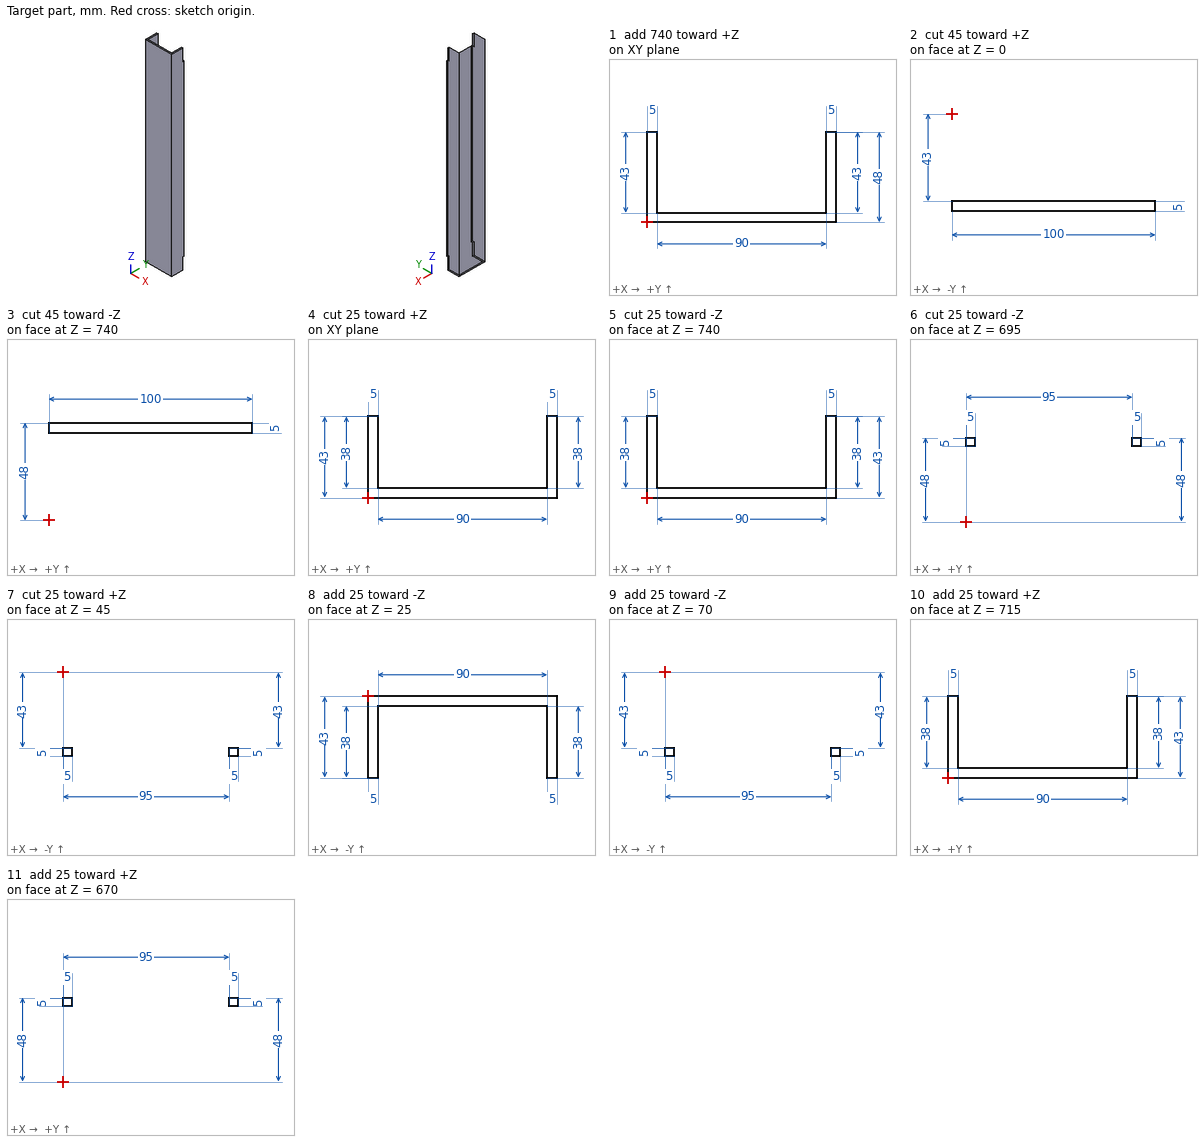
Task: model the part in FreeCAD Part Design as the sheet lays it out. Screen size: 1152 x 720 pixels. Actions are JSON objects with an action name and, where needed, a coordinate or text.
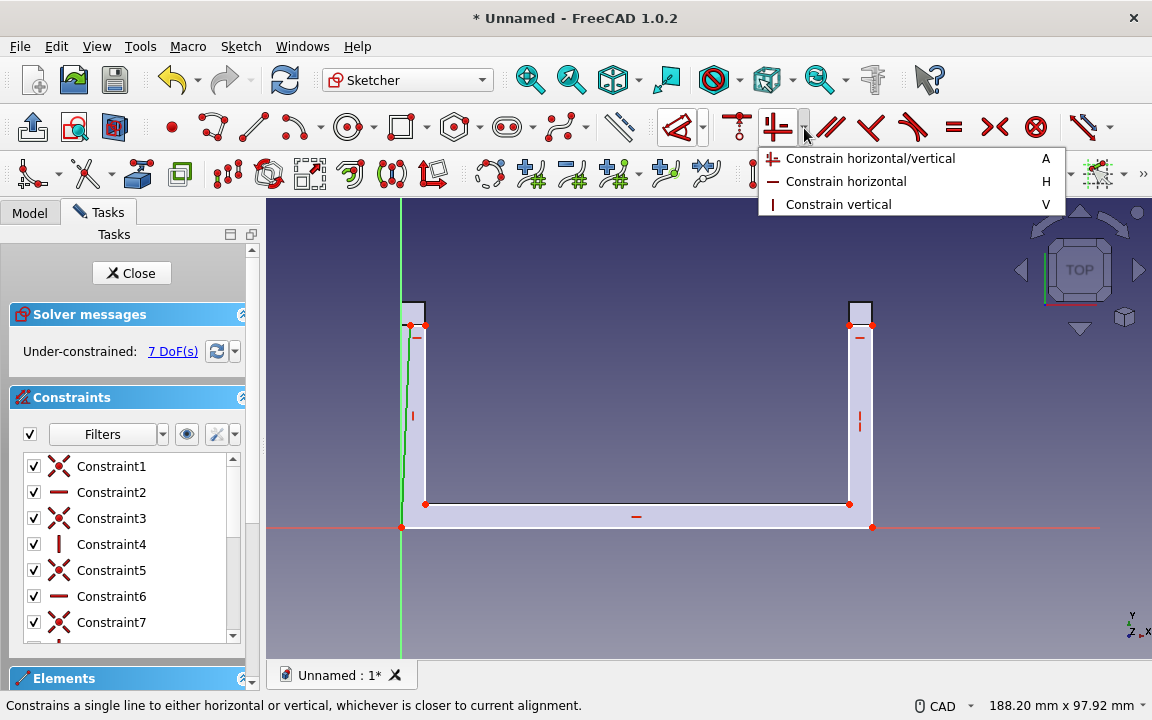
{"action": "left_click", "coordinate": [912, 204]}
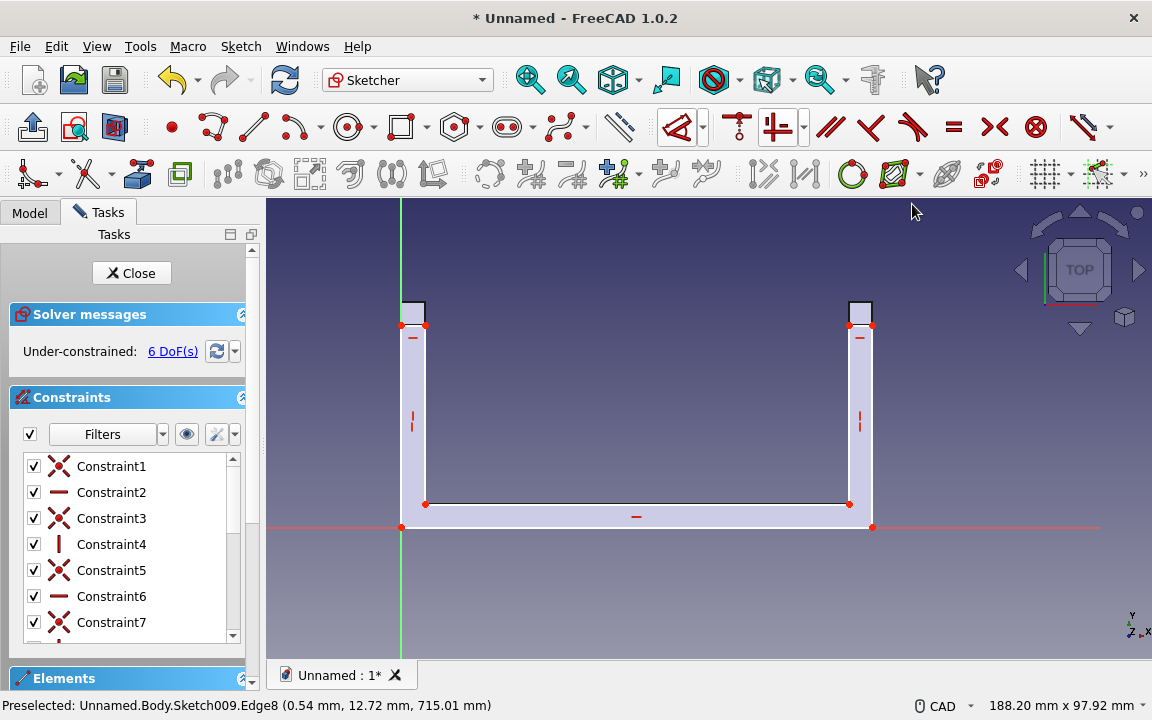
{"action": "scroll", "coordinate": [863, 326], "scroll_direction": "up", "scroll_amount": 3}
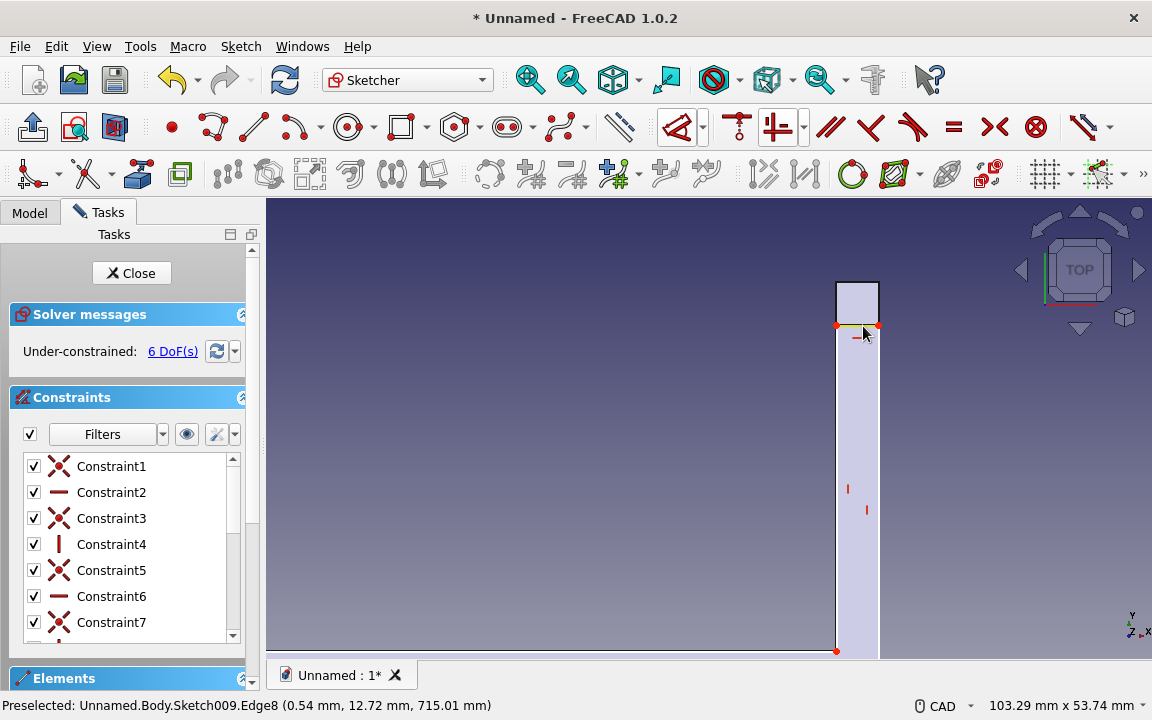
{"action": "left_click", "coordinate": [862, 326]}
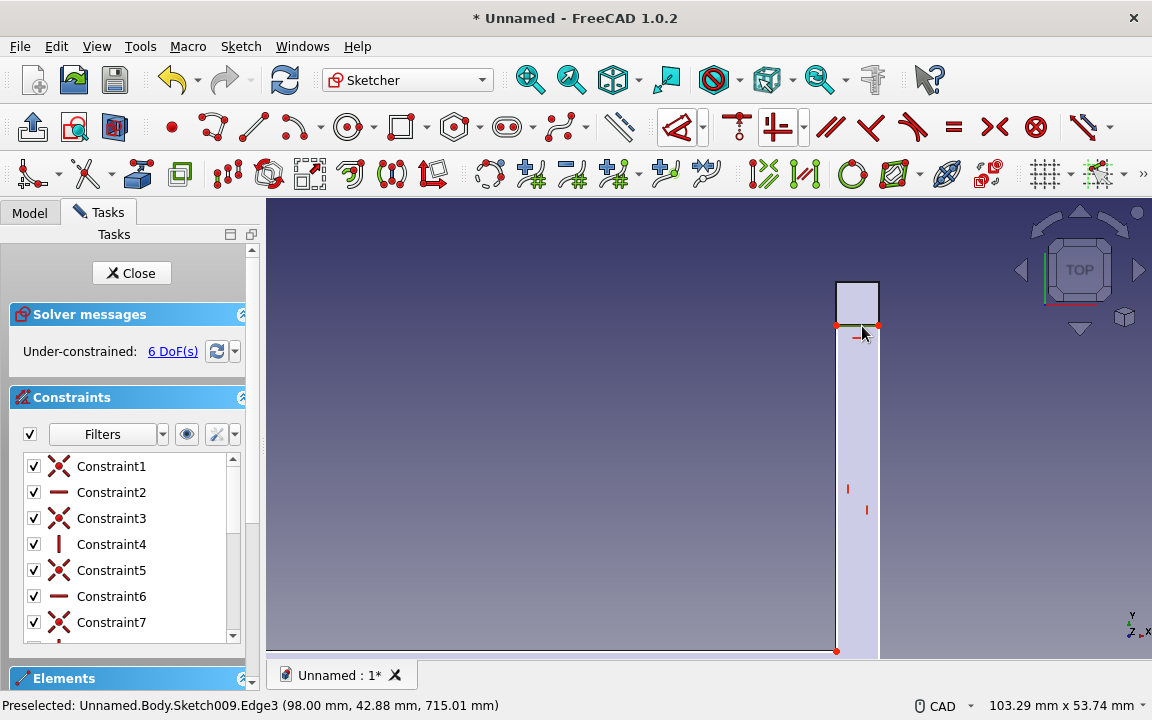
{"action": "left_click", "coordinate": [702, 128]}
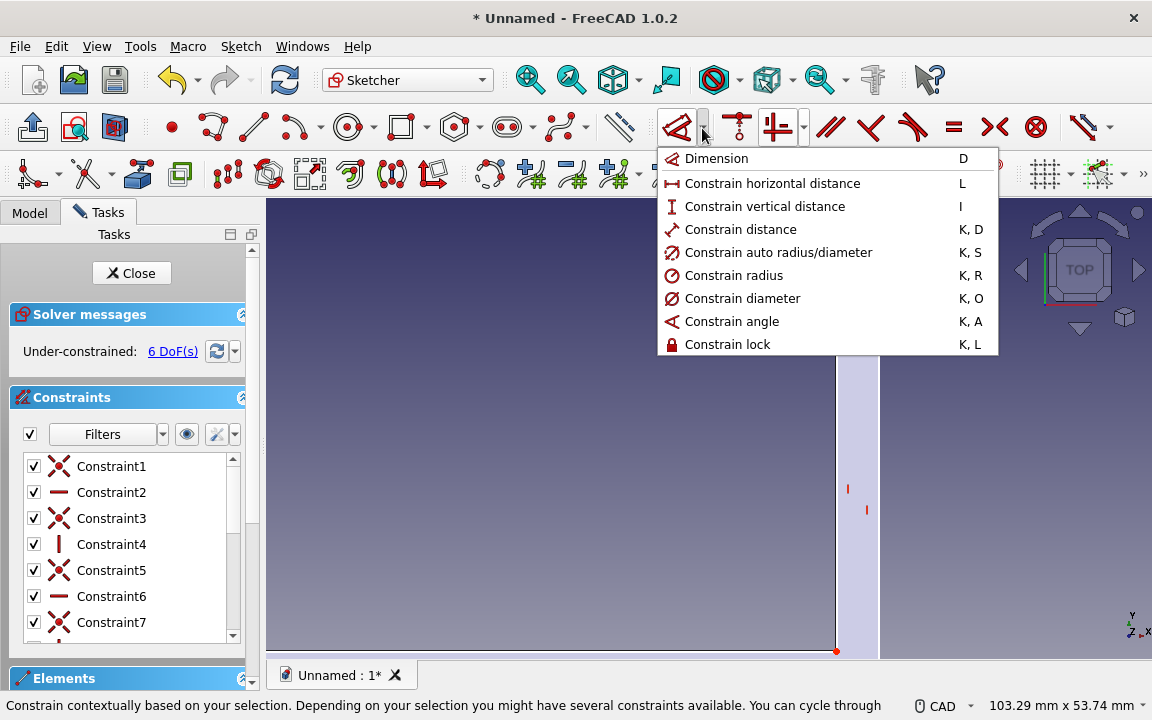
{"action": "left_click", "coordinate": [828, 184]}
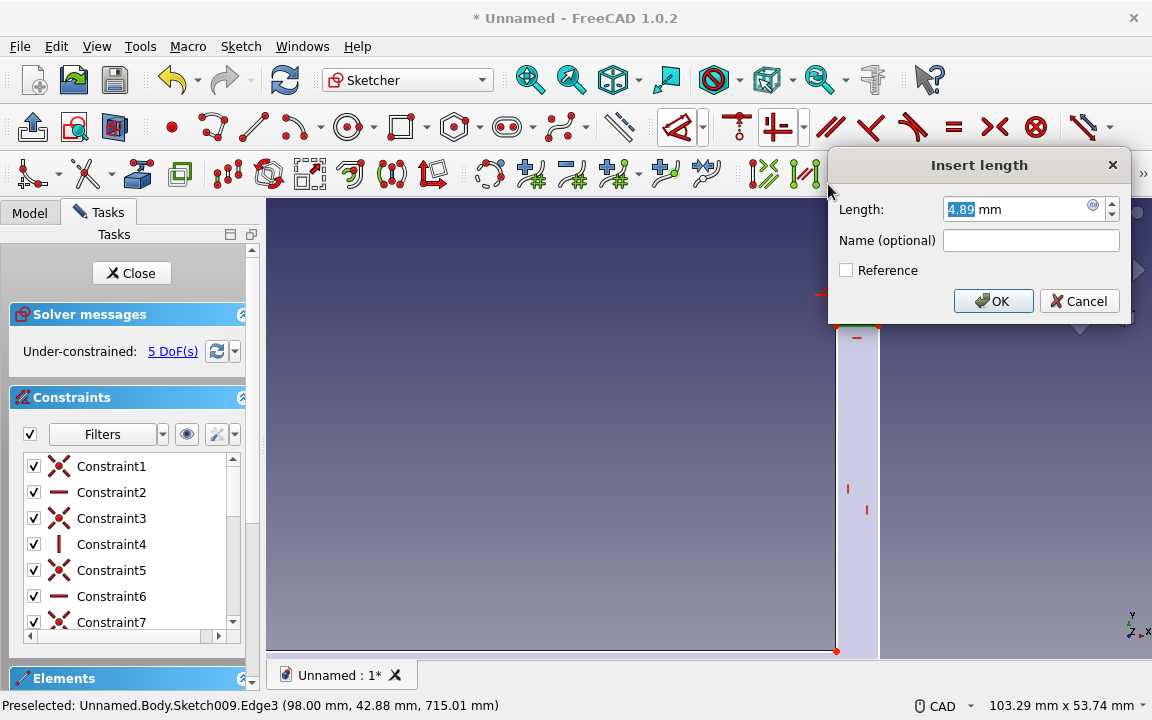
{"action": "type", "text": "5"}
{"action": "key", "text": "Return"}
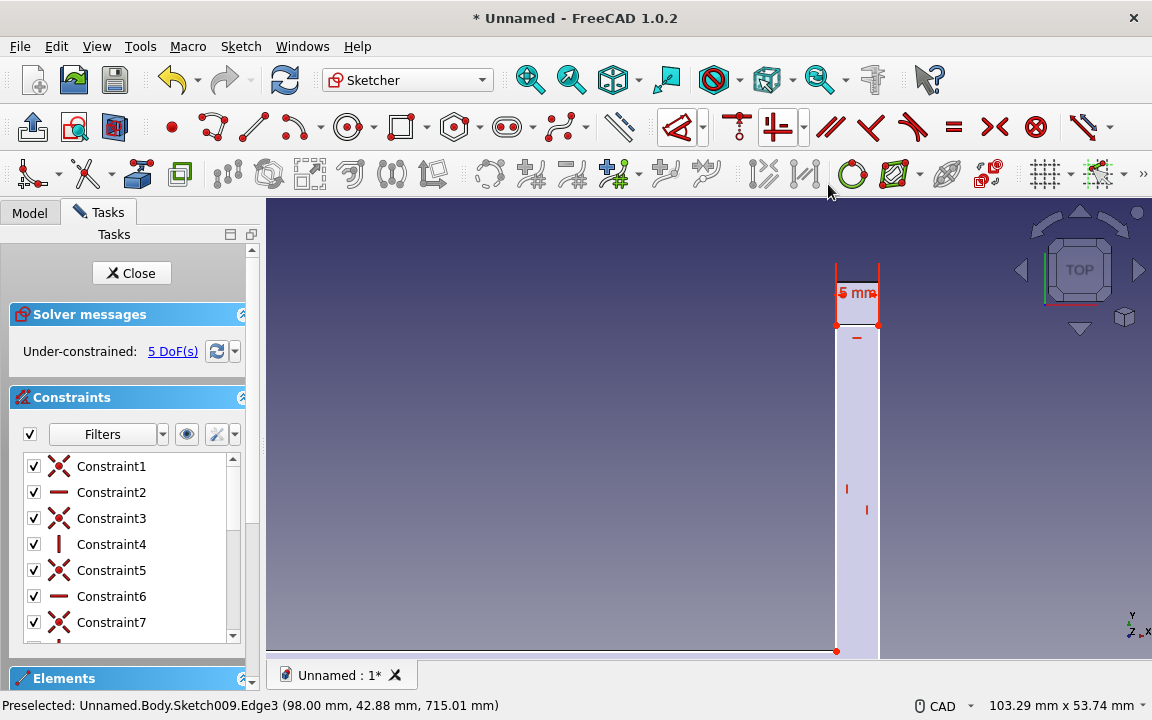
{"action": "scroll", "coordinate": [872, 330], "scroll_direction": "down", "scroll_amount": 3}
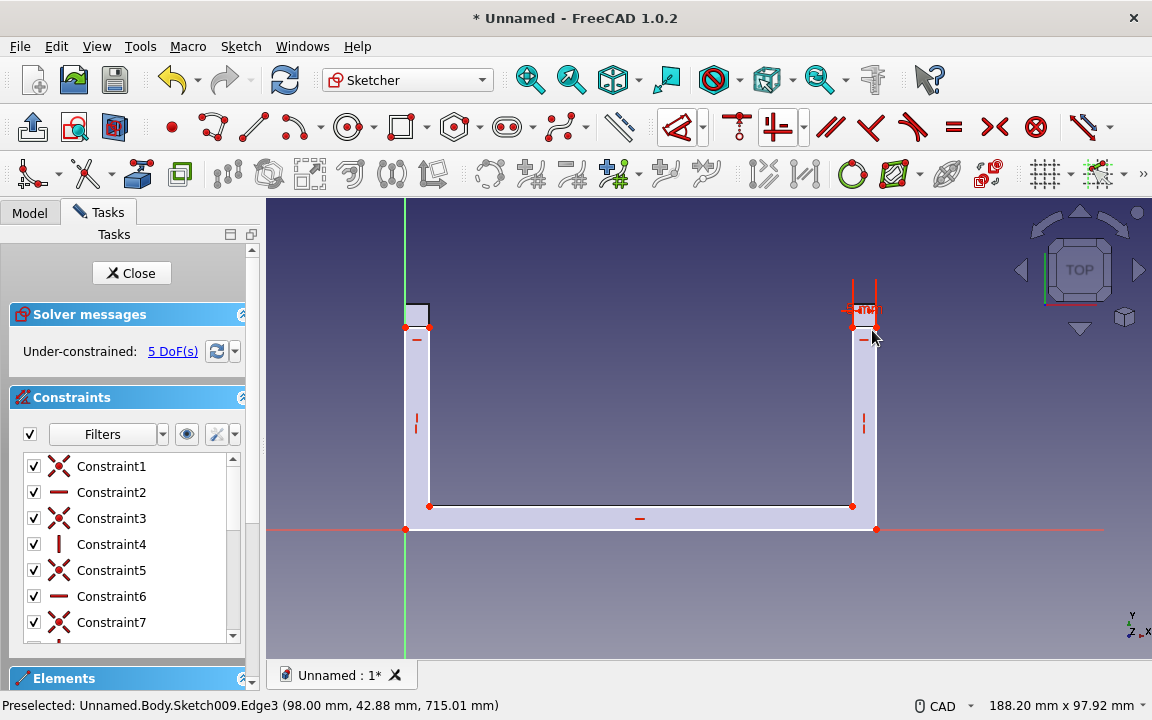
{"action": "scroll", "coordinate": [422, 328], "scroll_direction": "up", "scroll_amount": 4}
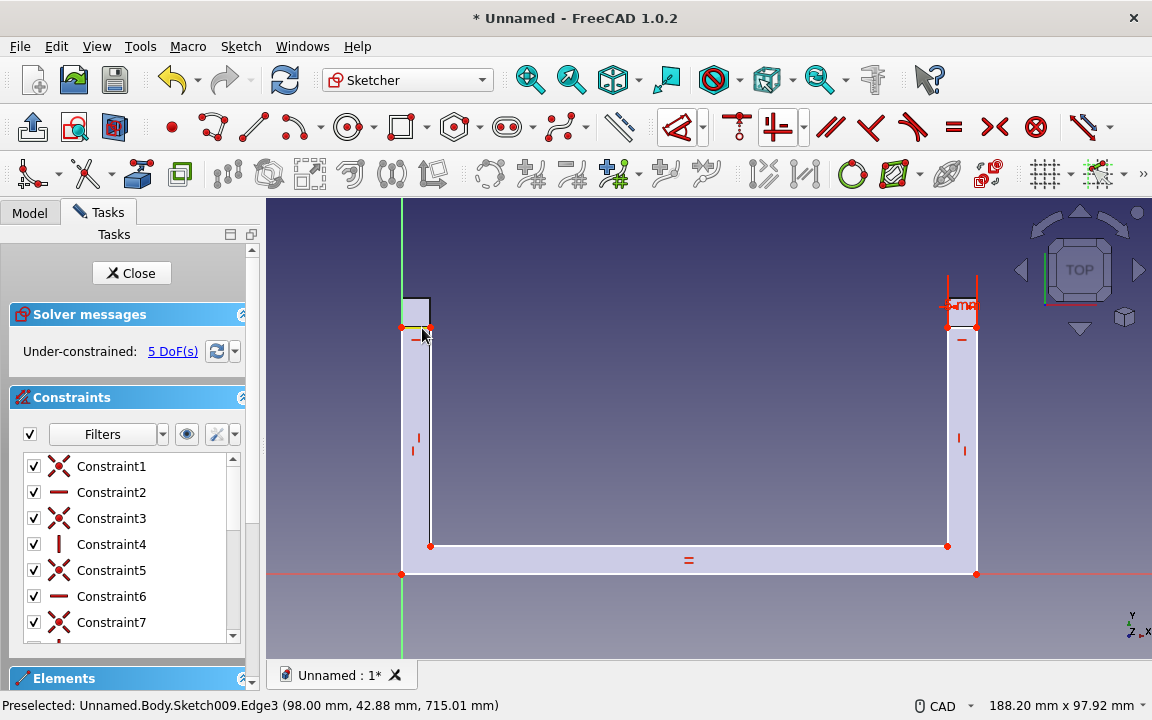
{"action": "left_click", "coordinate": [422, 327]}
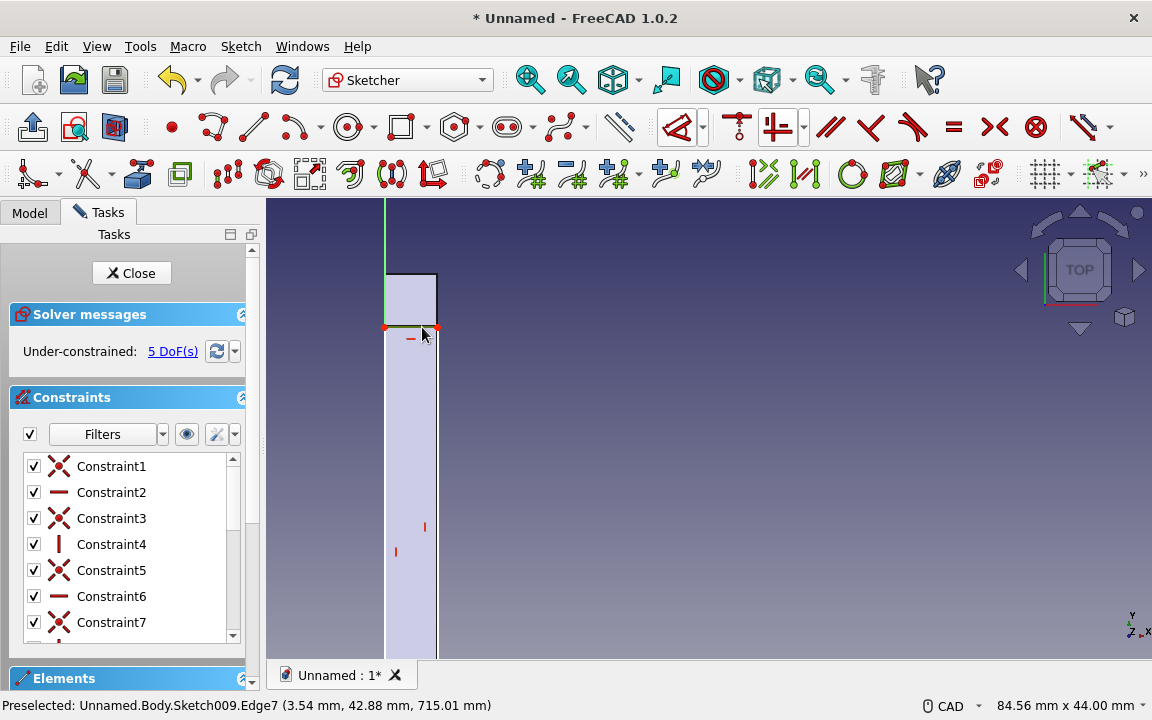
{"action": "left_click", "coordinate": [702, 128]}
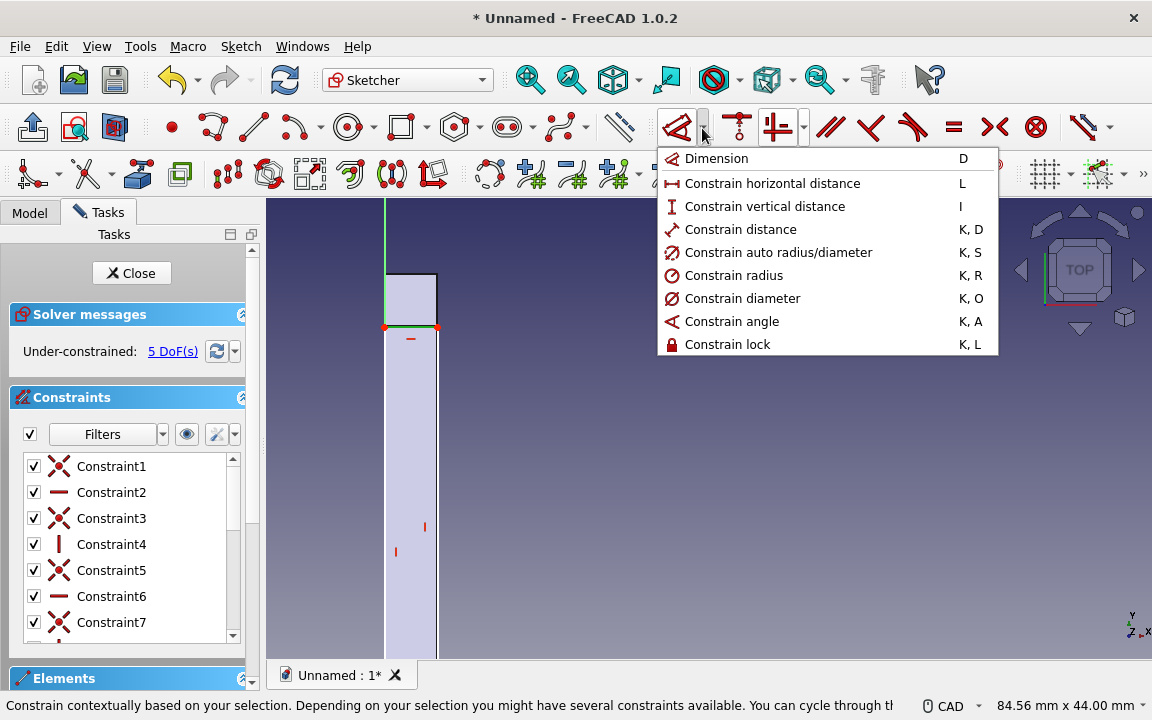
{"action": "left_click", "coordinate": [828, 184]}